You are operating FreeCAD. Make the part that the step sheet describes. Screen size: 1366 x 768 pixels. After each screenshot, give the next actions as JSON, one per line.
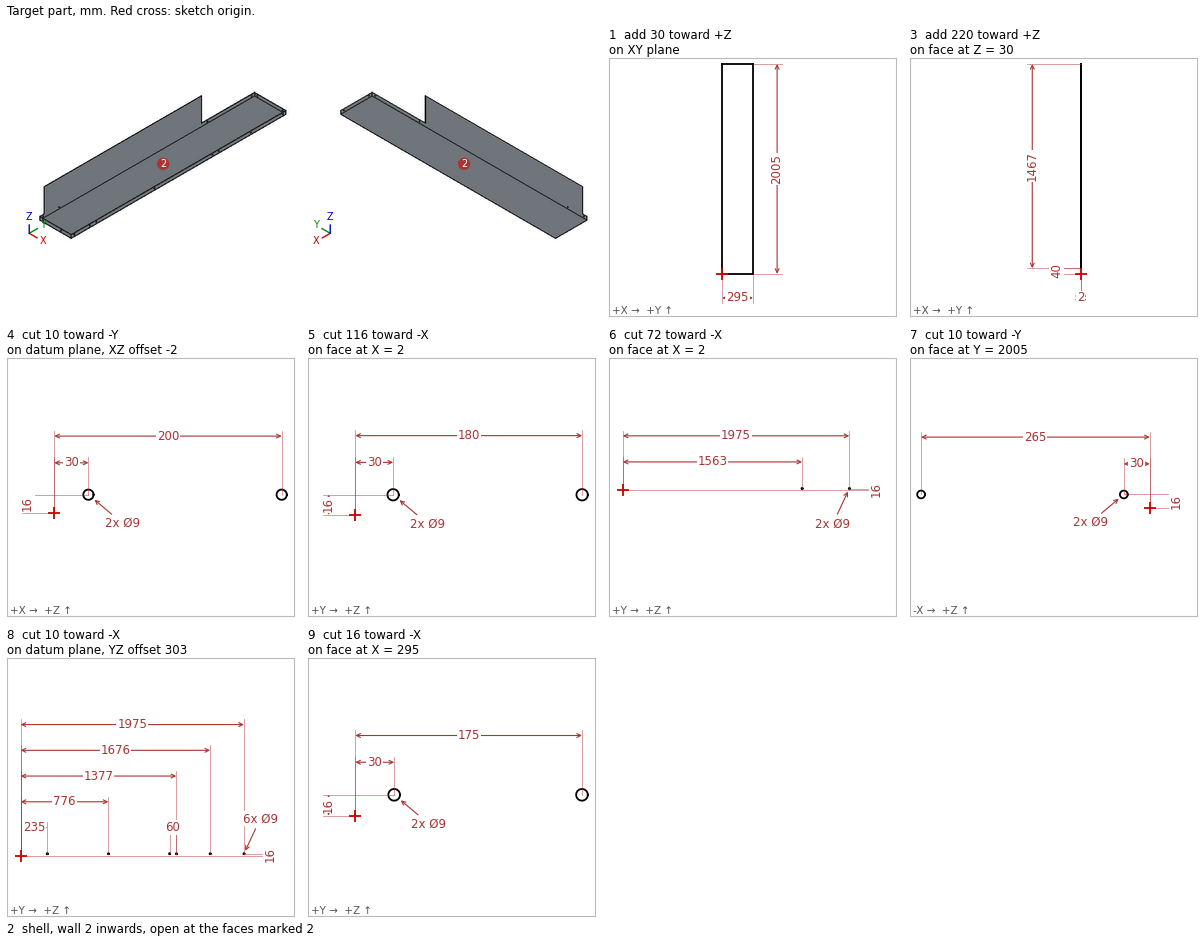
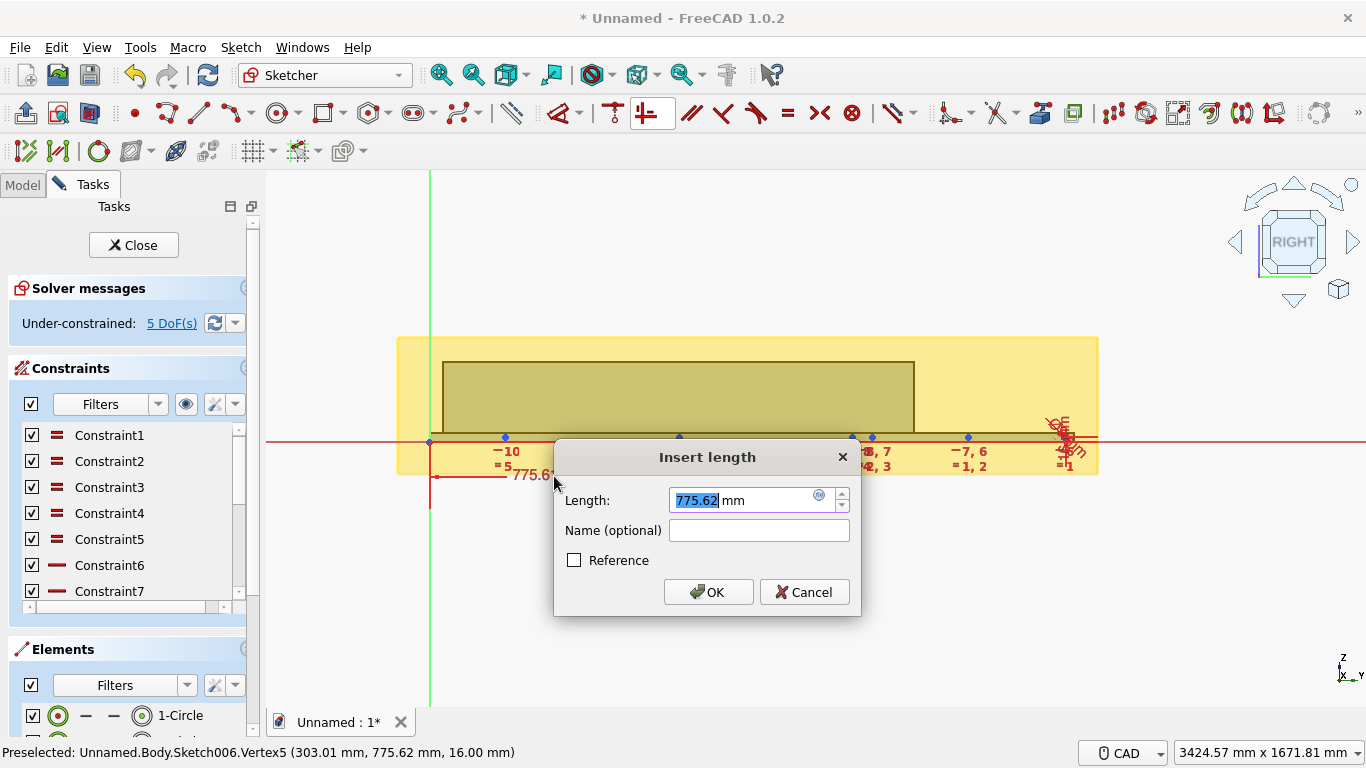
{"action": "type", "text": "776"}
{"action": "key", "text": "Return"}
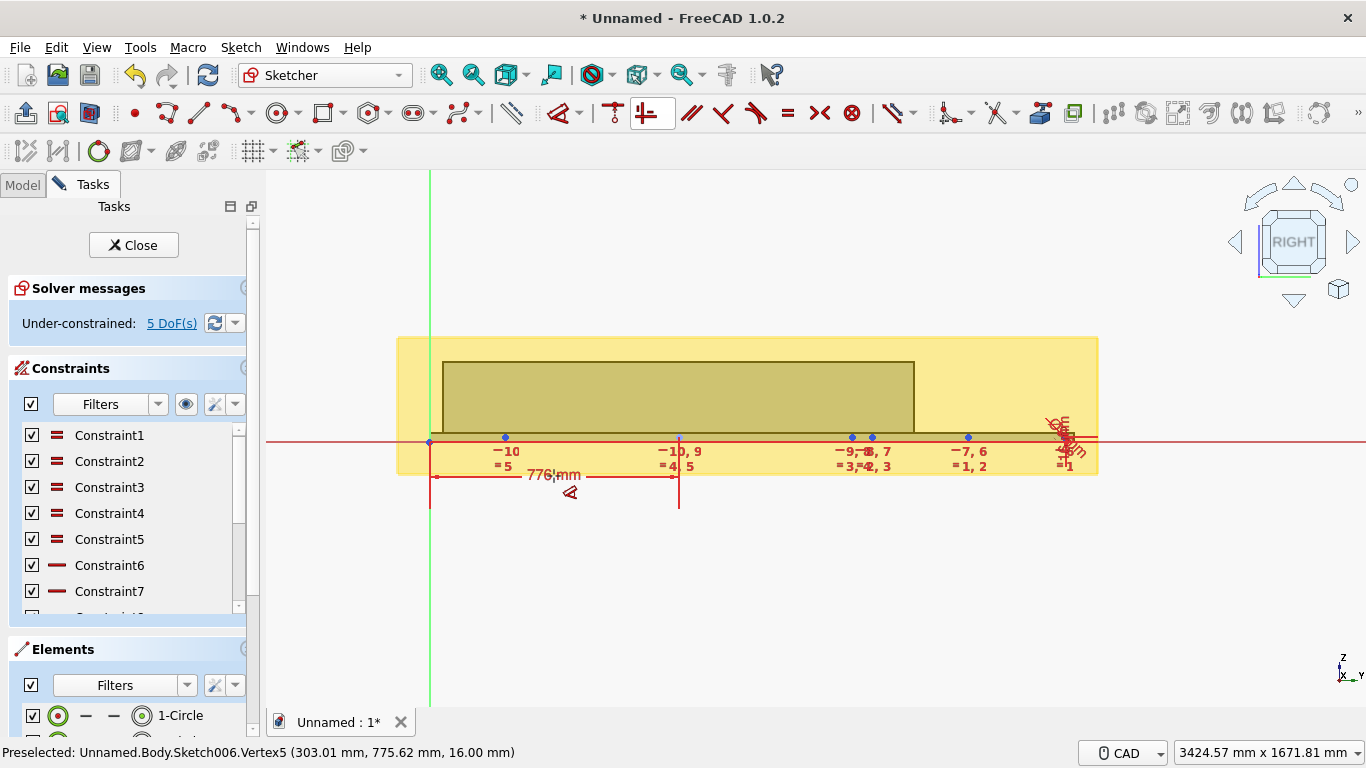
{"action": "left_click", "coordinate": [505, 437]}
{"action": "left_click", "coordinate": [468, 476]}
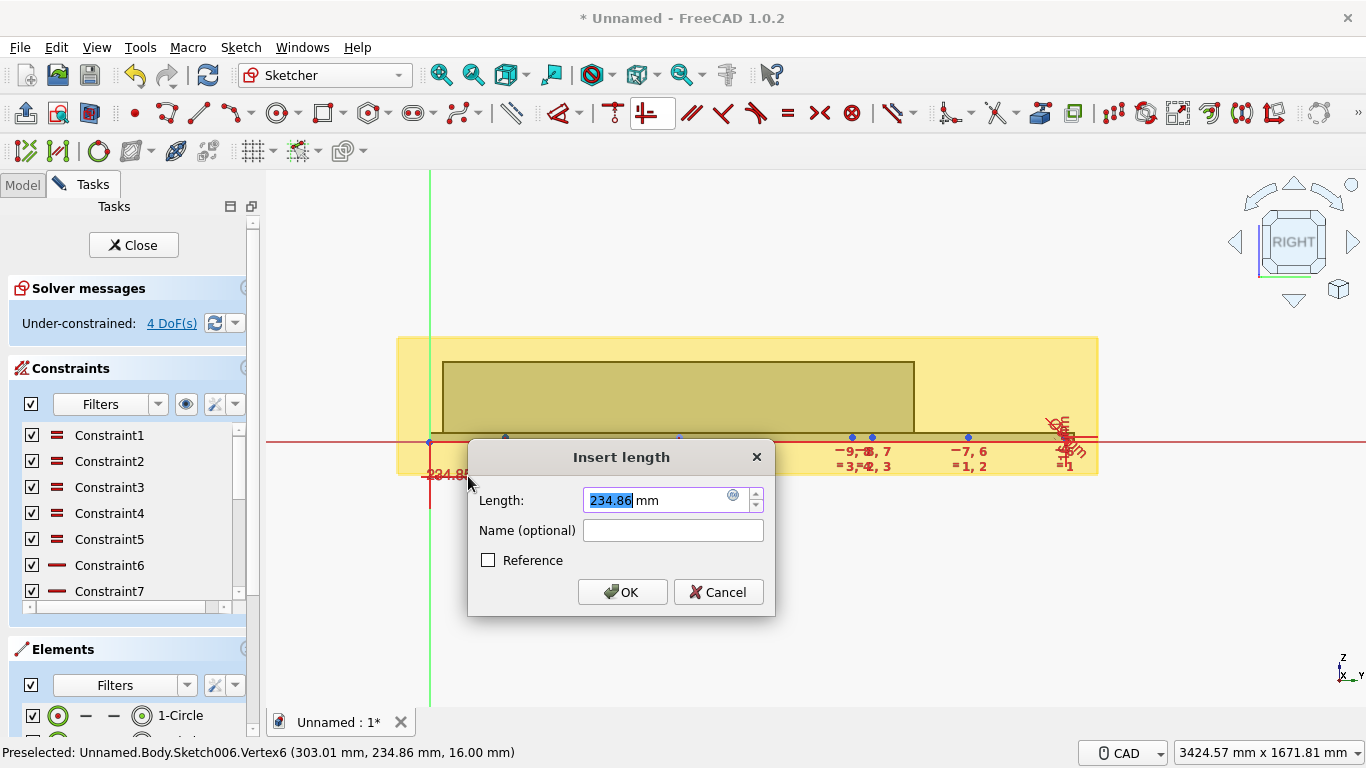
{"action": "type", "text": "235"}
{"action": "key", "text": "Return"}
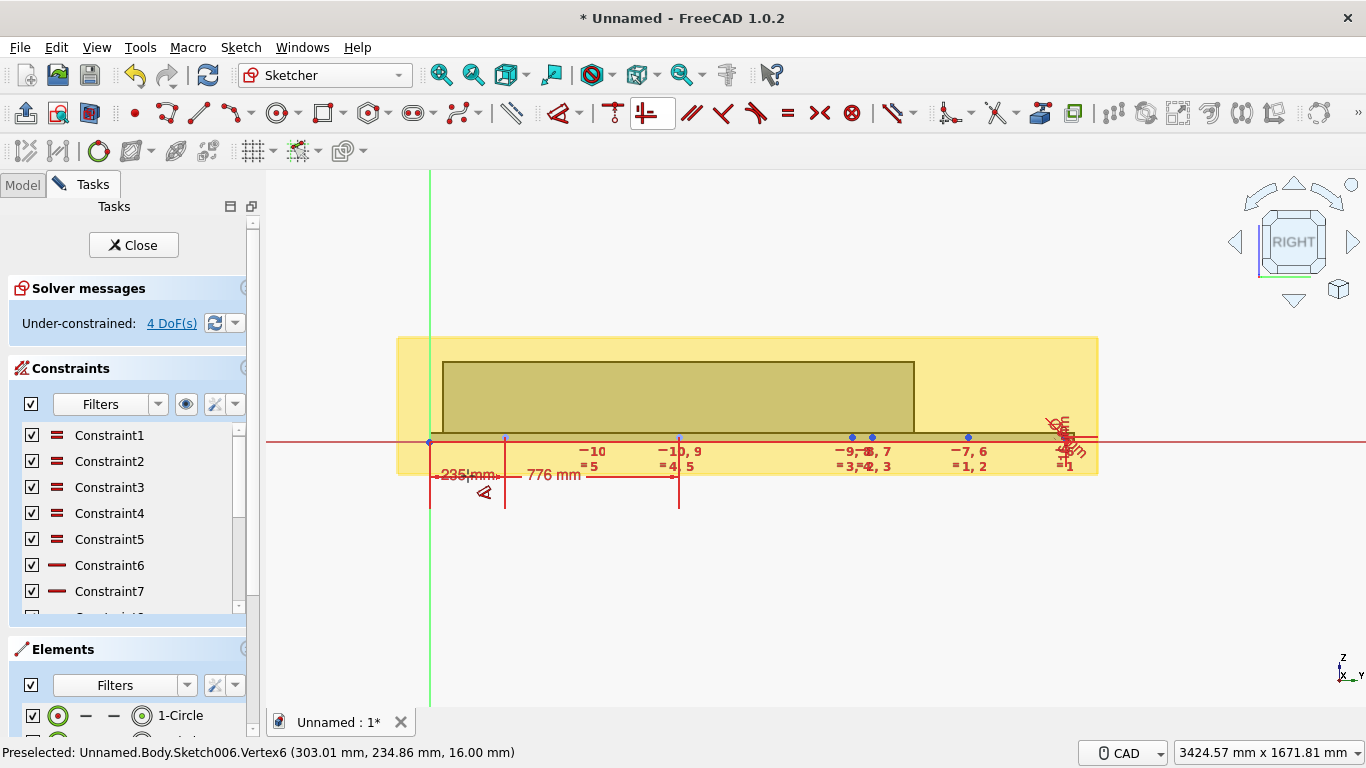
{"action": "scroll", "coordinate": [872, 437], "scroll_direction": "up", "scroll_amount": 4}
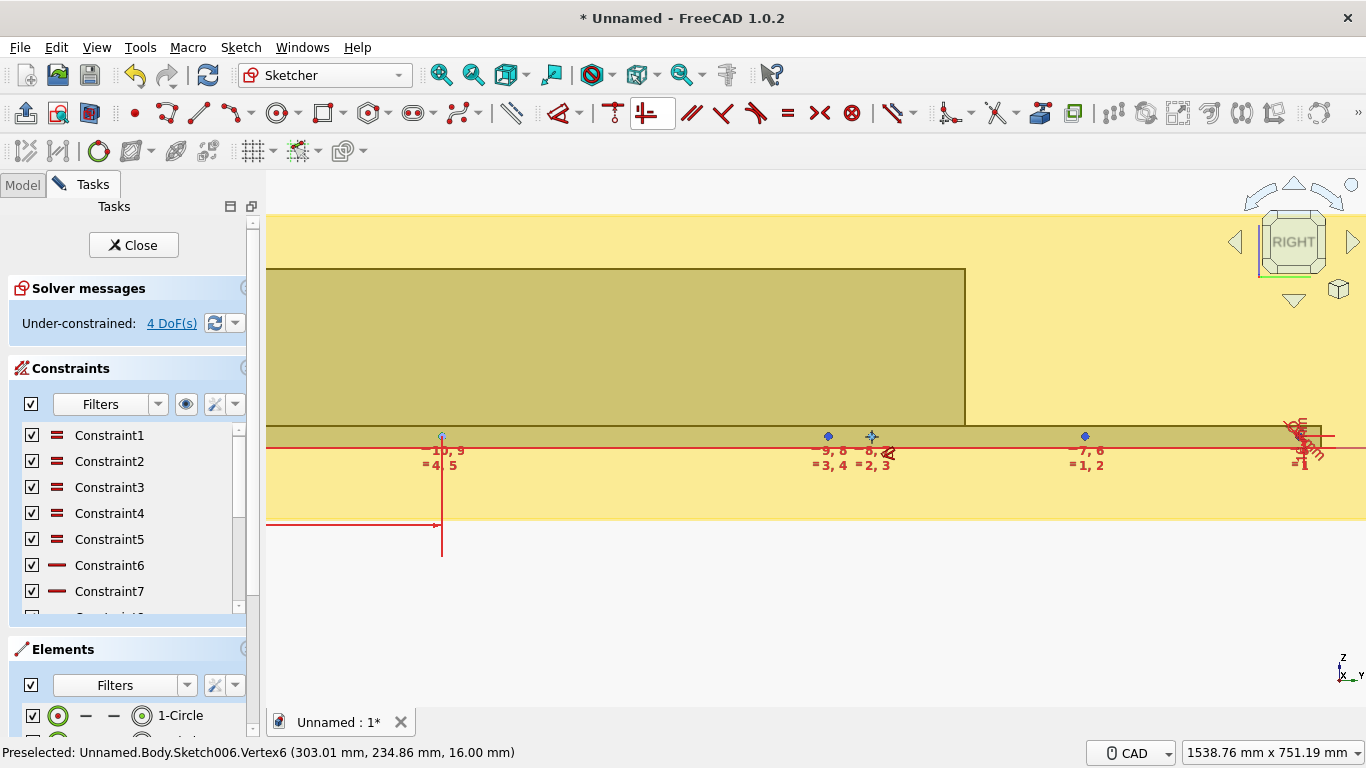
{"action": "left_click", "coordinate": [872, 436]}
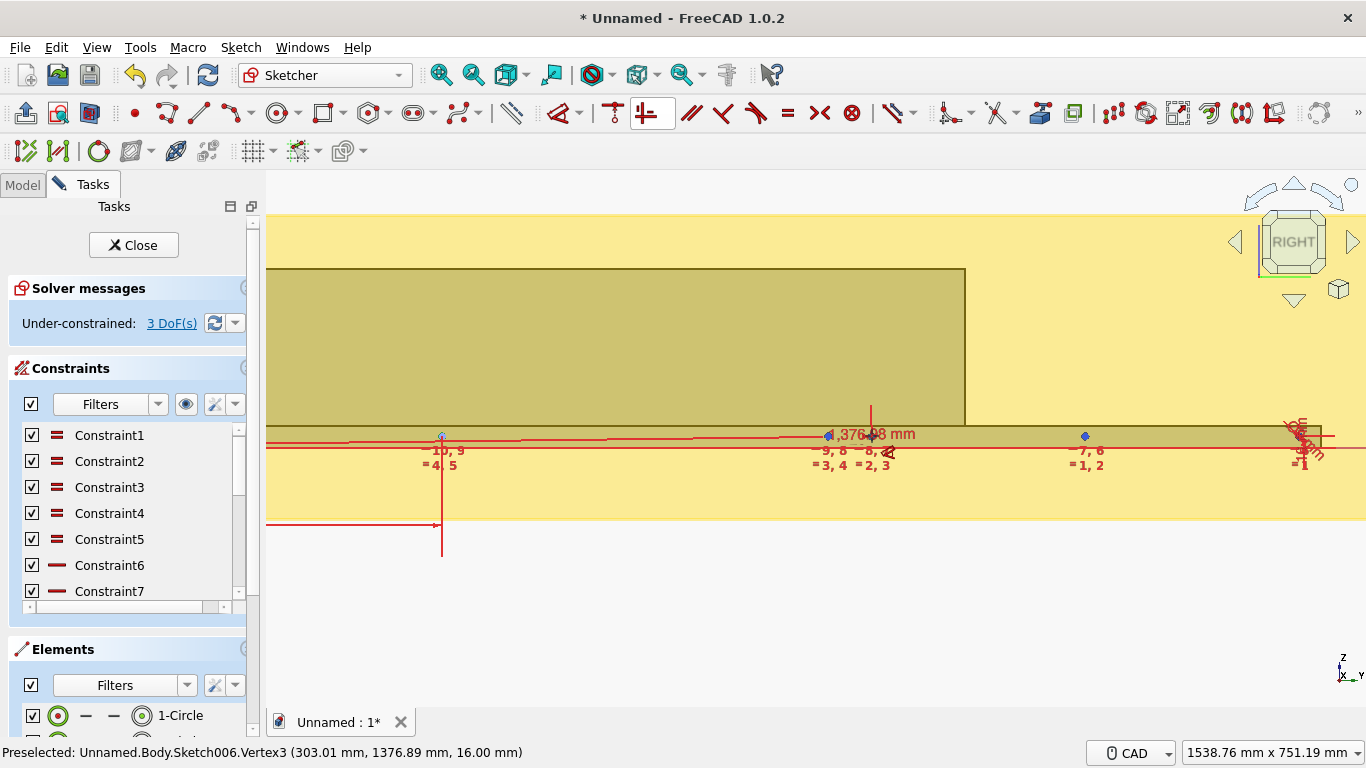
{"action": "left_click", "coordinate": [828, 436]}
{"action": "left_click", "coordinate": [850, 402]}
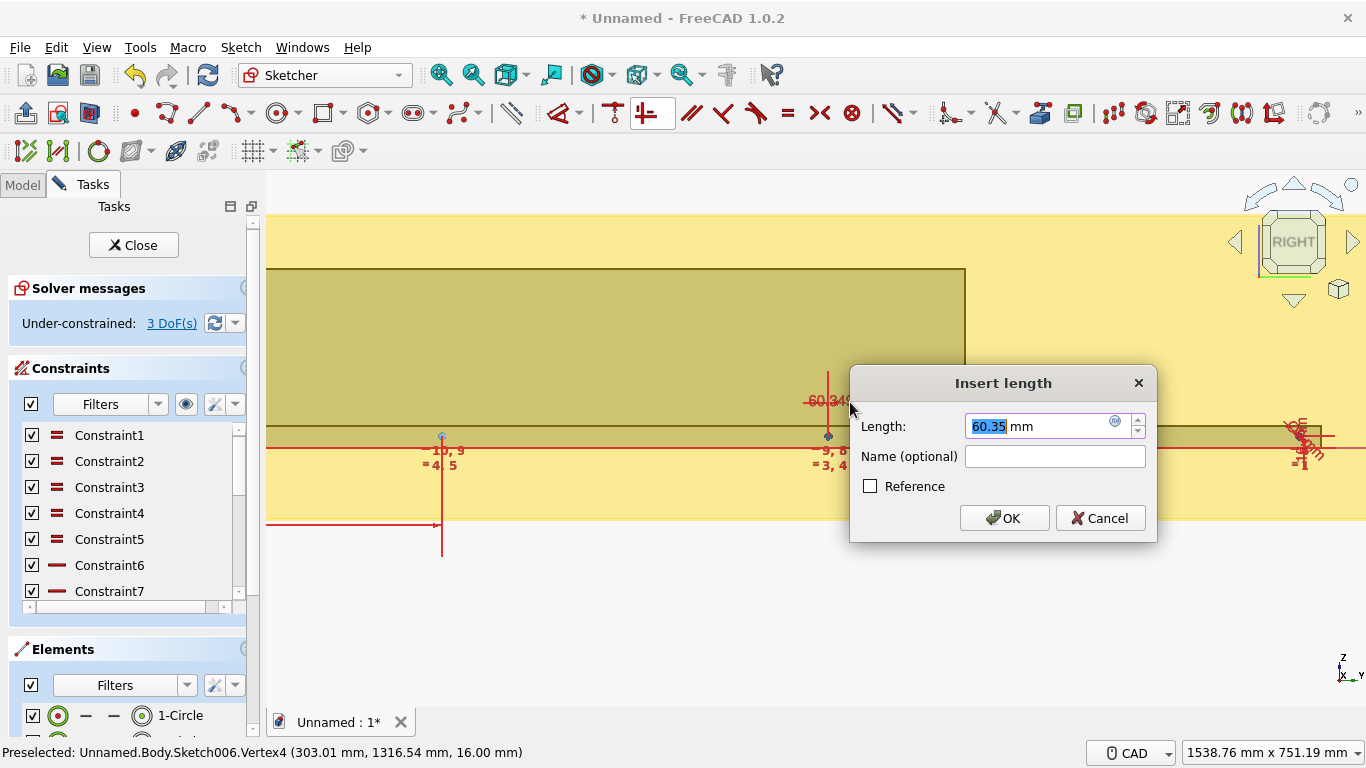
{"action": "type", "text": "60"}
{"action": "key", "text": "Return"}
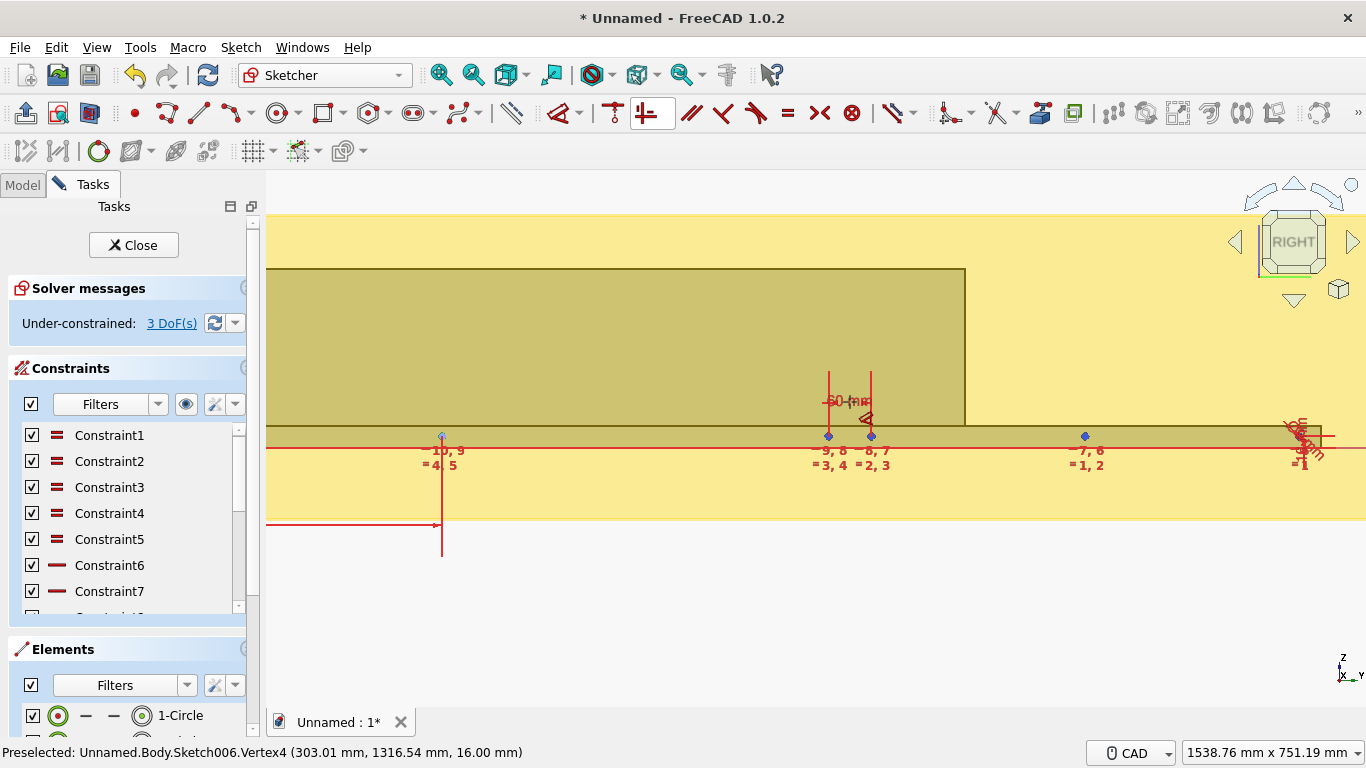
{"action": "scroll", "coordinate": [872, 437], "scroll_direction": "down", "scroll_amount": 4}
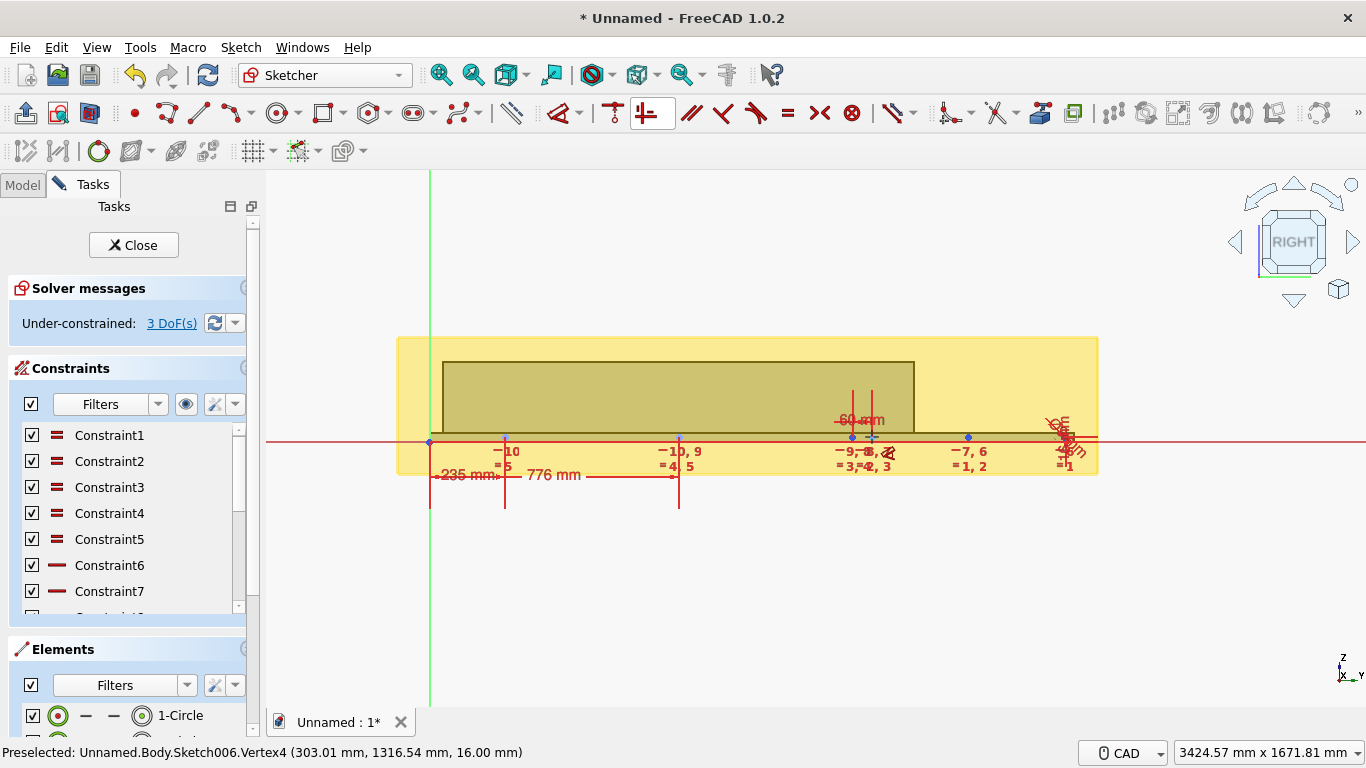
{"action": "left_click", "coordinate": [1064, 437]}
{"action": "left_click", "coordinate": [747, 476]}